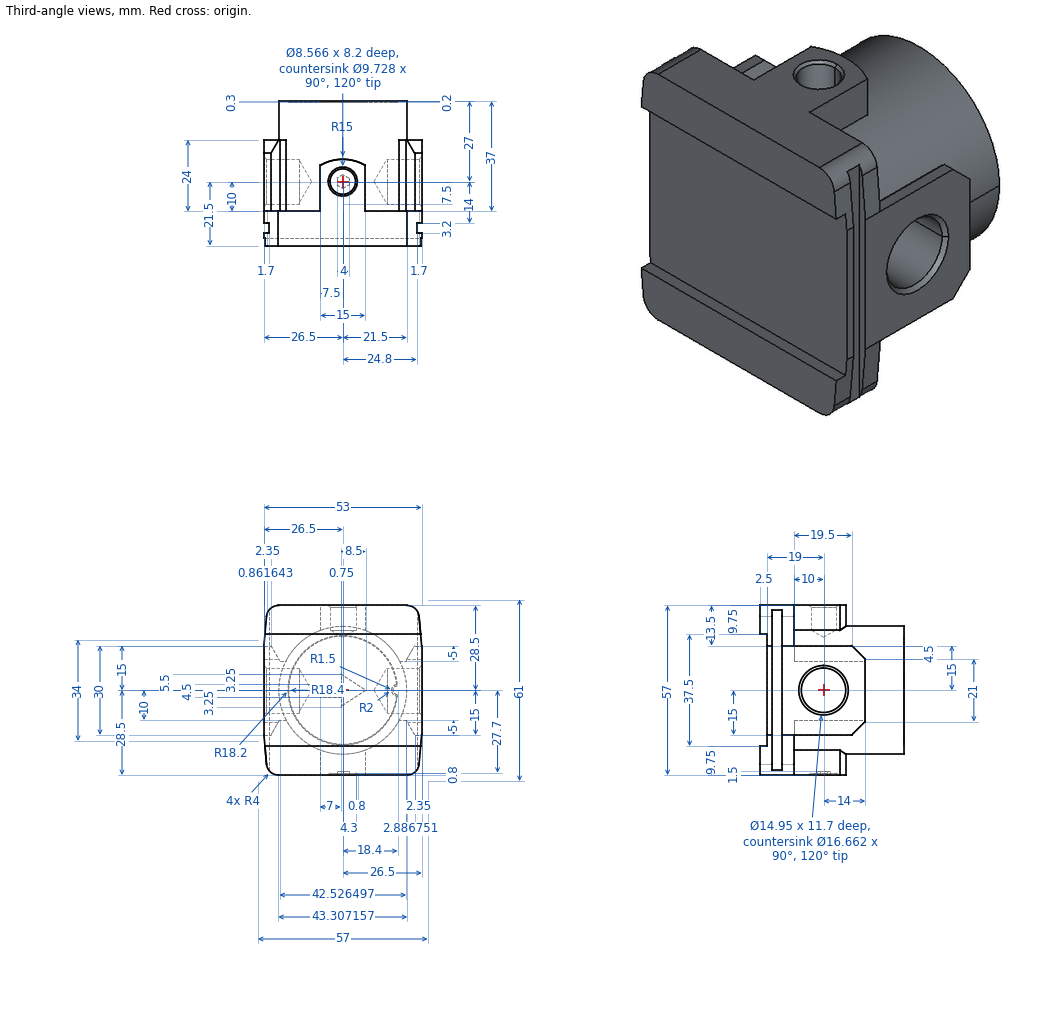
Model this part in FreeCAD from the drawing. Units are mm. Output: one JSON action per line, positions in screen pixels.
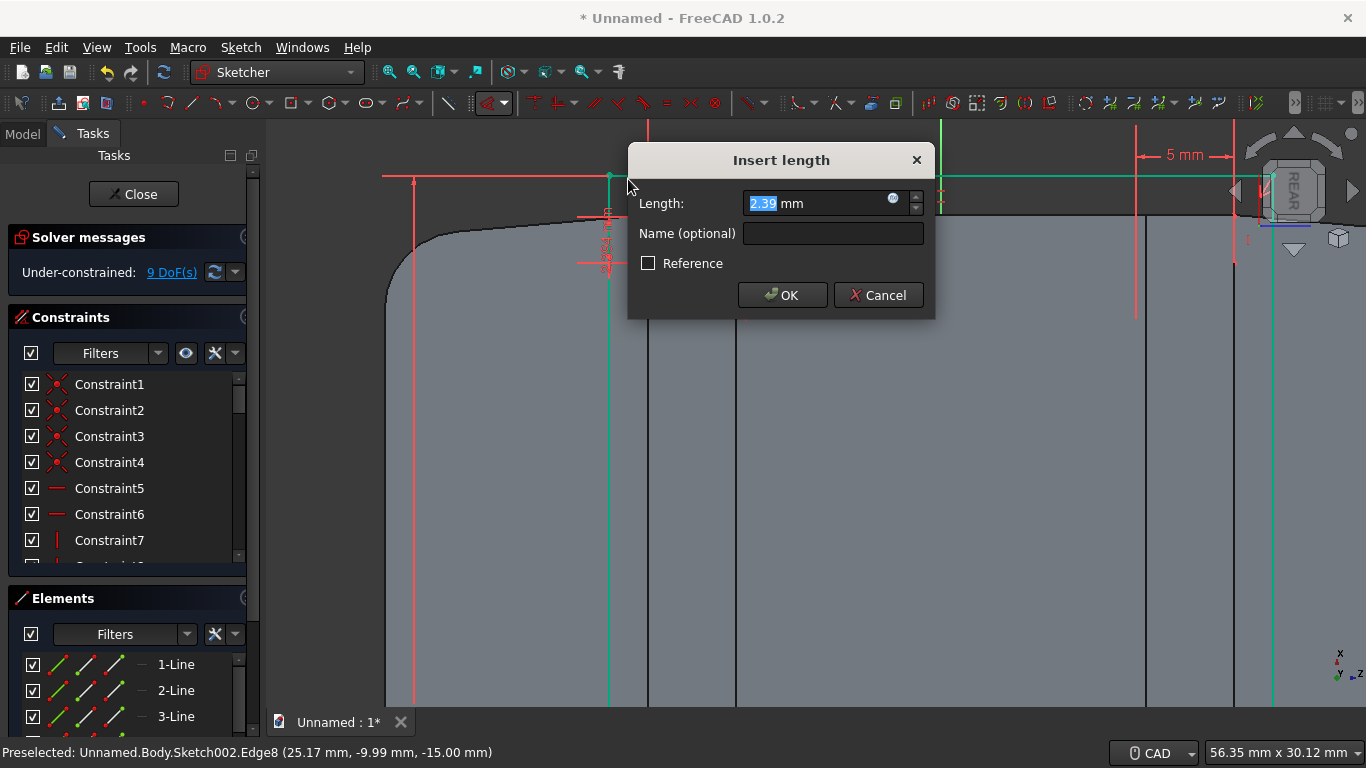
{"action": "type", "text": "2.35"}
{"action": "key", "text": "Return"}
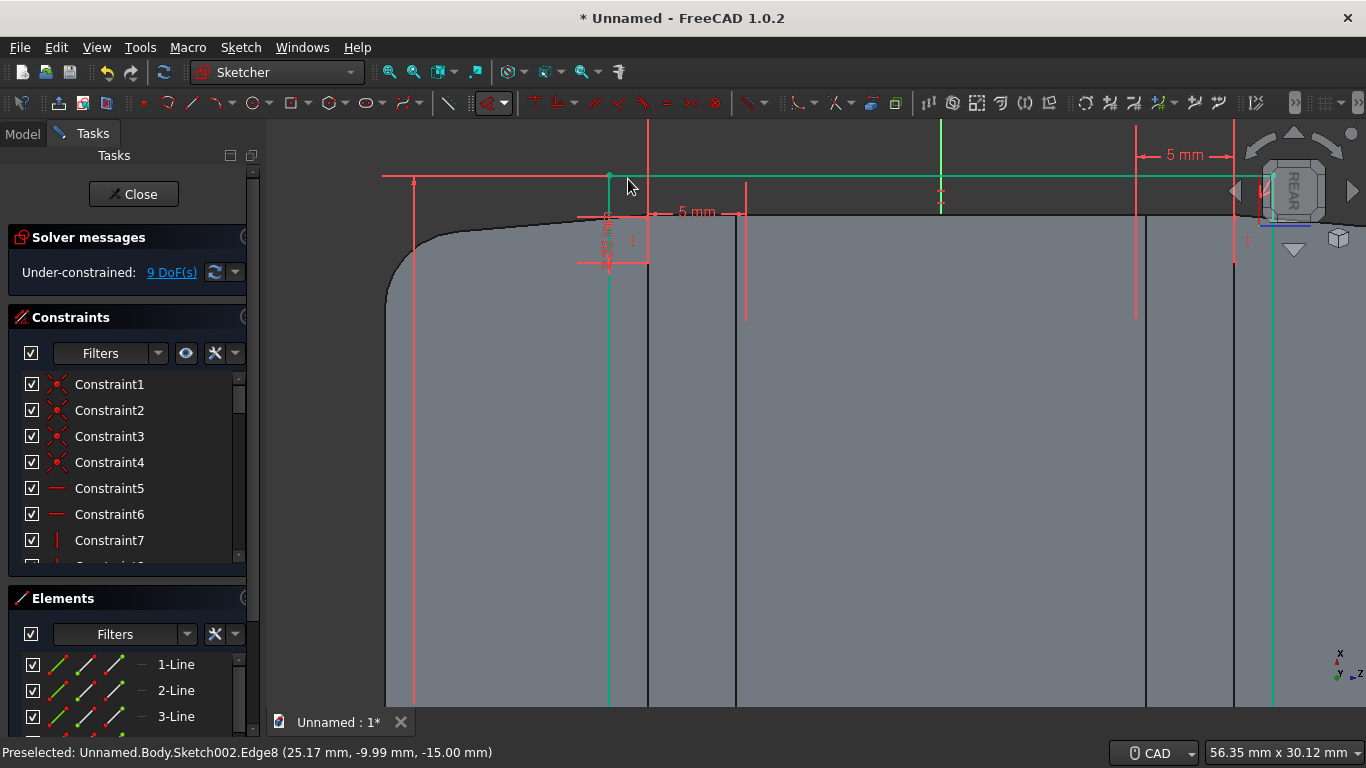
{"action": "scroll", "coordinate": [635, 227], "scroll_direction": "down", "scroll_amount": 5}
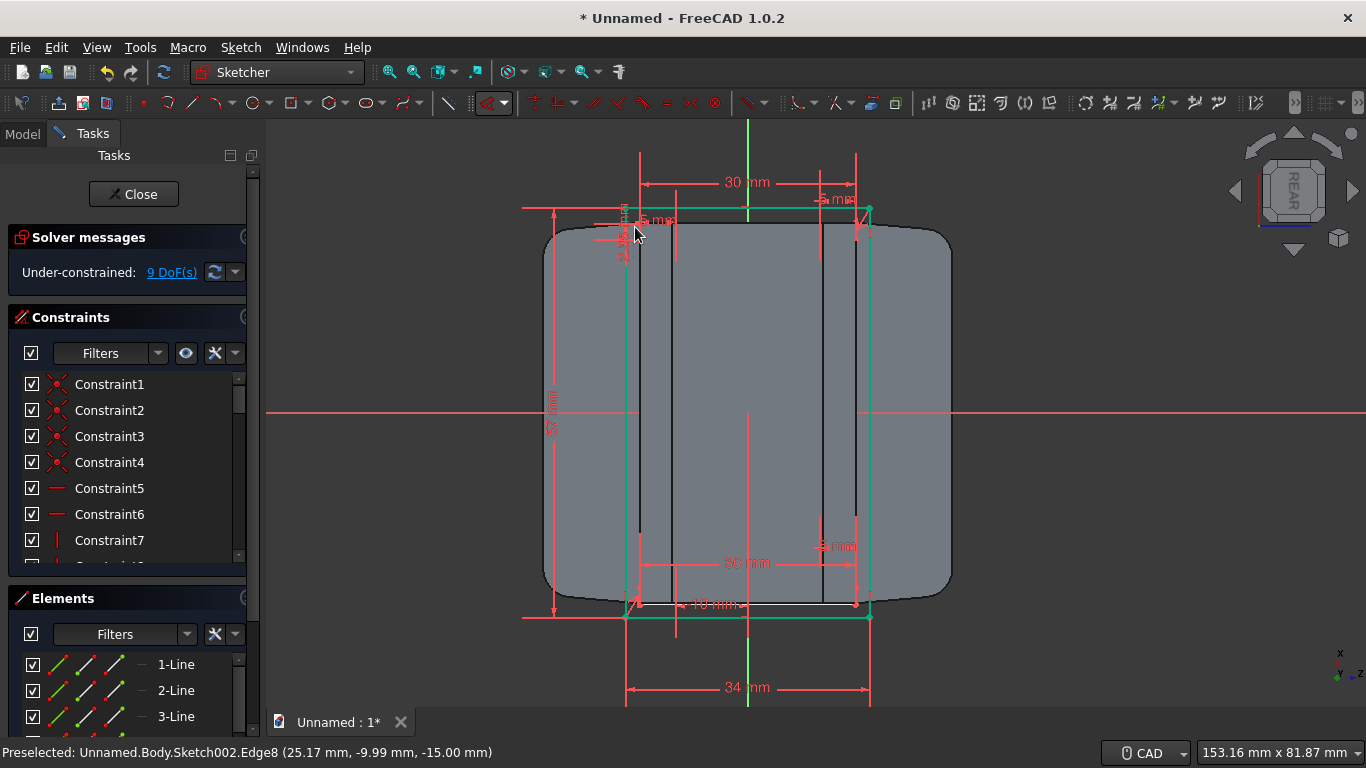
{"action": "scroll", "coordinate": [856, 229], "scroll_direction": "up", "scroll_amount": 6}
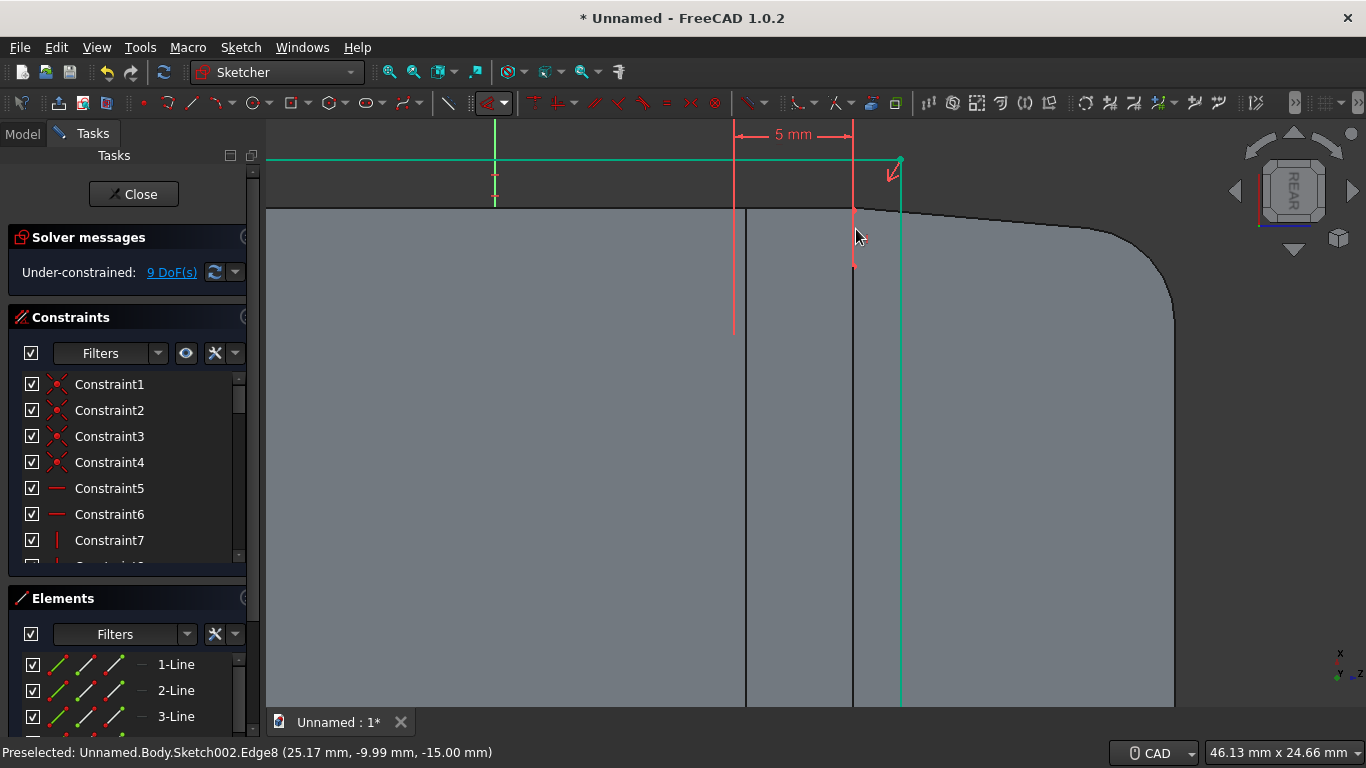
{"action": "left_click", "coordinate": [853, 227]}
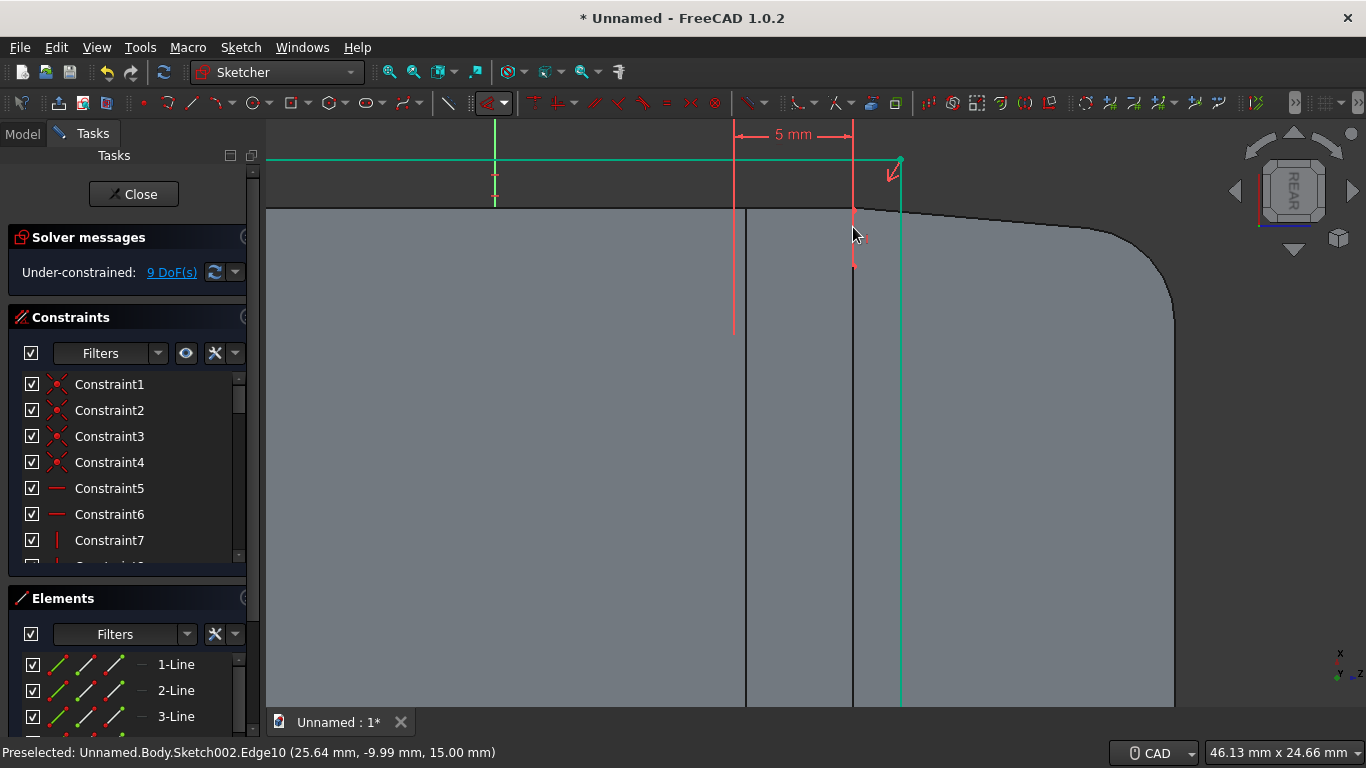
{"action": "key", "text": "i"}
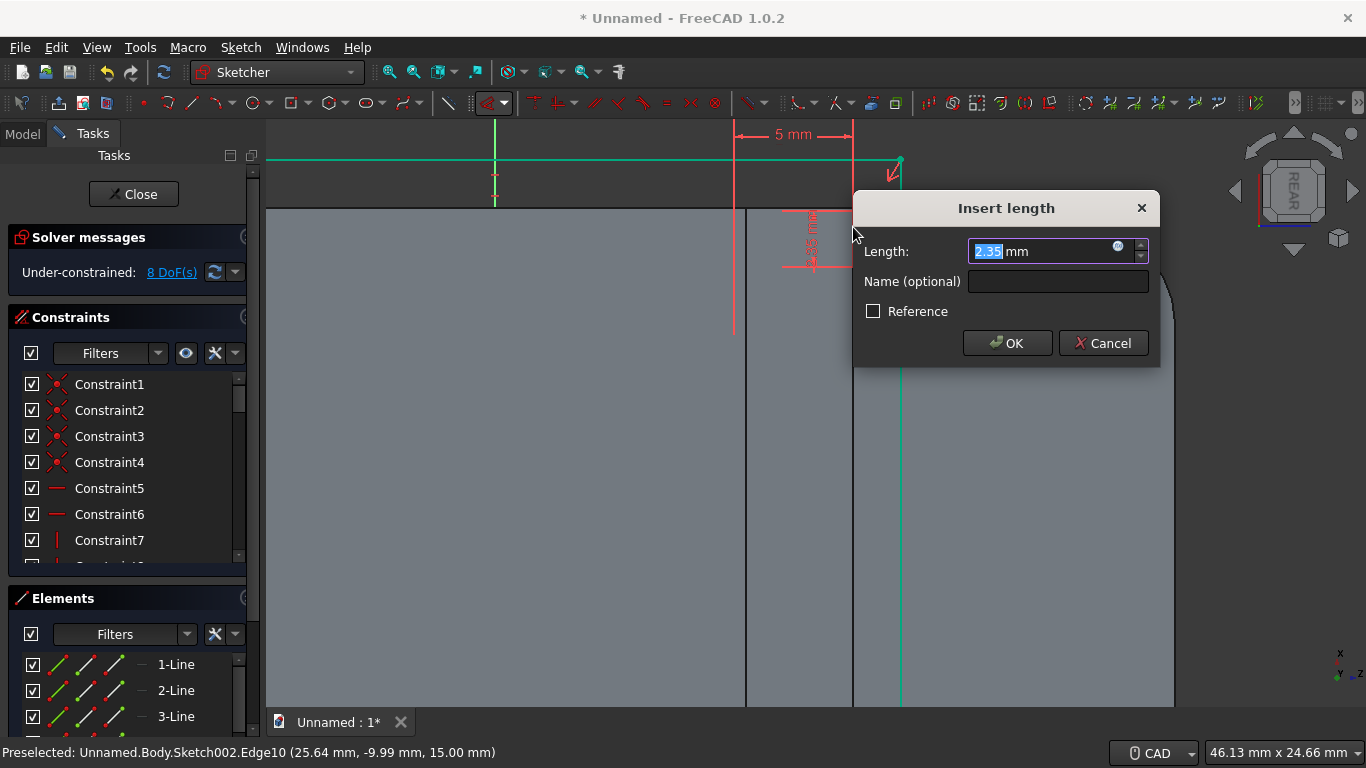
{"action": "type", "text": "2.35"}
{"action": "key", "text": "Return"}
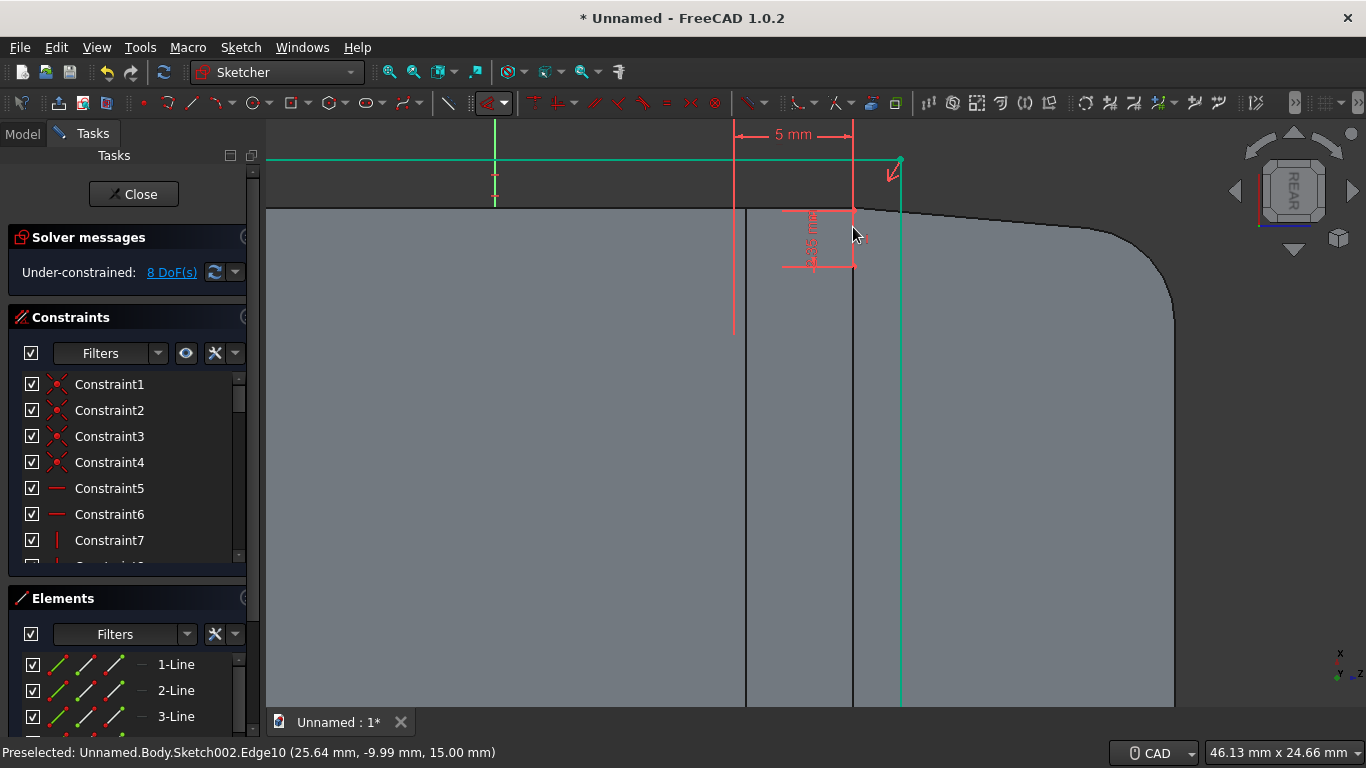
{"action": "scroll", "coordinate": [856, 229], "scroll_direction": "down", "scroll_amount": 6}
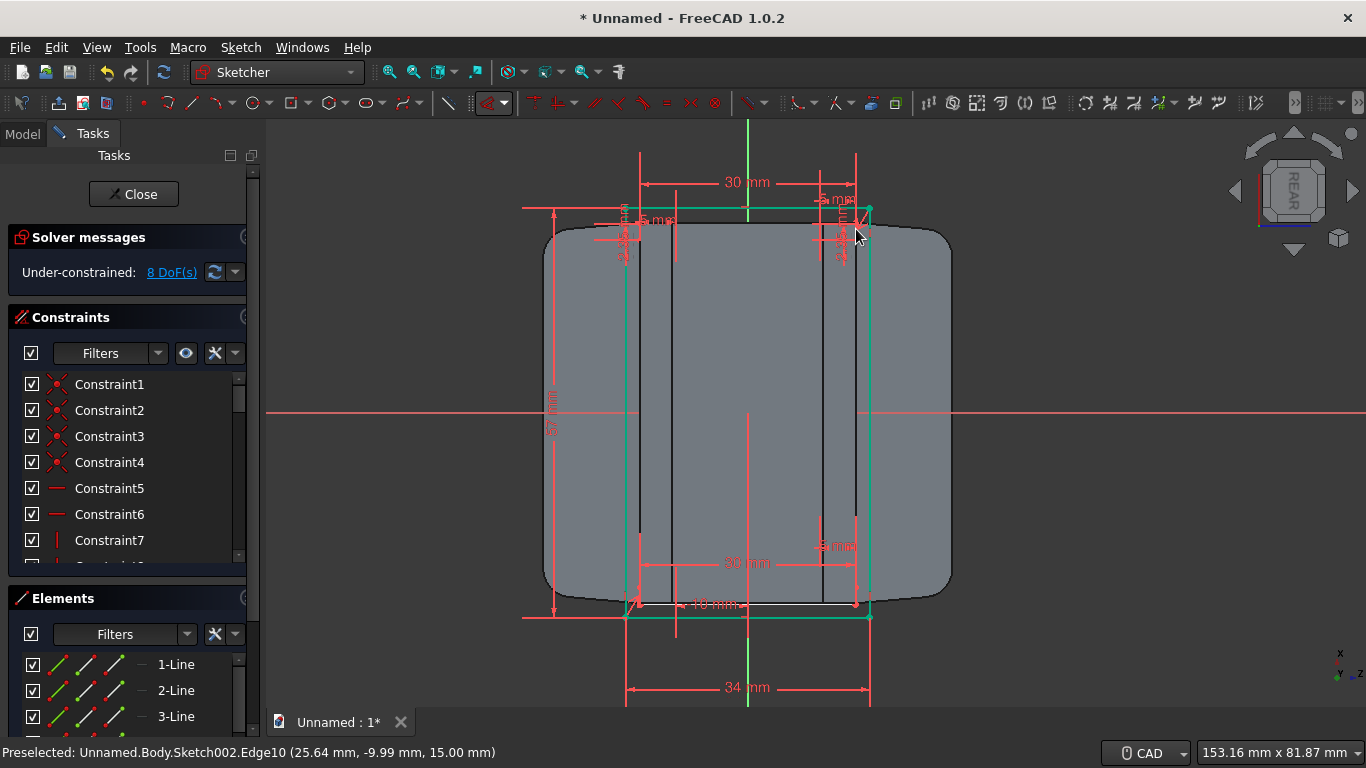
{"action": "scroll", "coordinate": [856, 592], "scroll_direction": "up", "scroll_amount": 5}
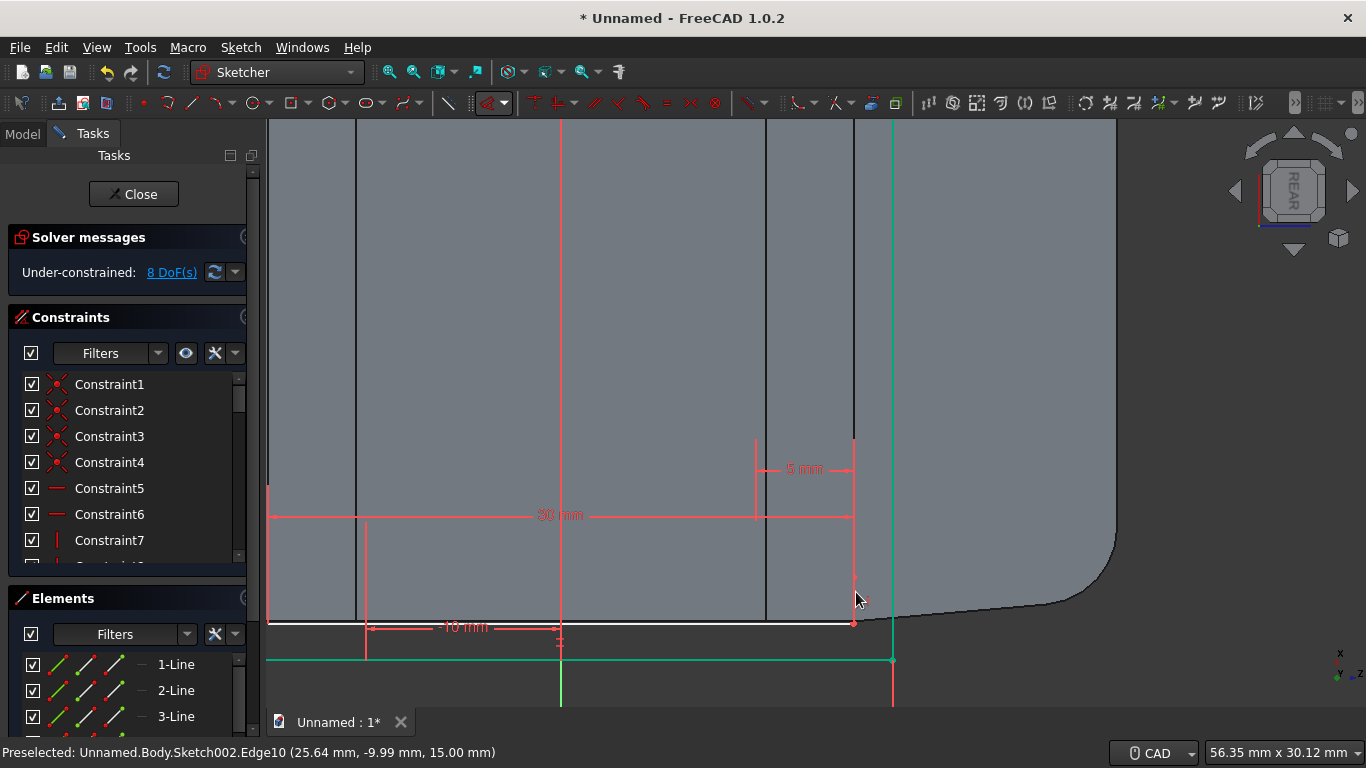
{"action": "left_click", "coordinate": [854, 591]}